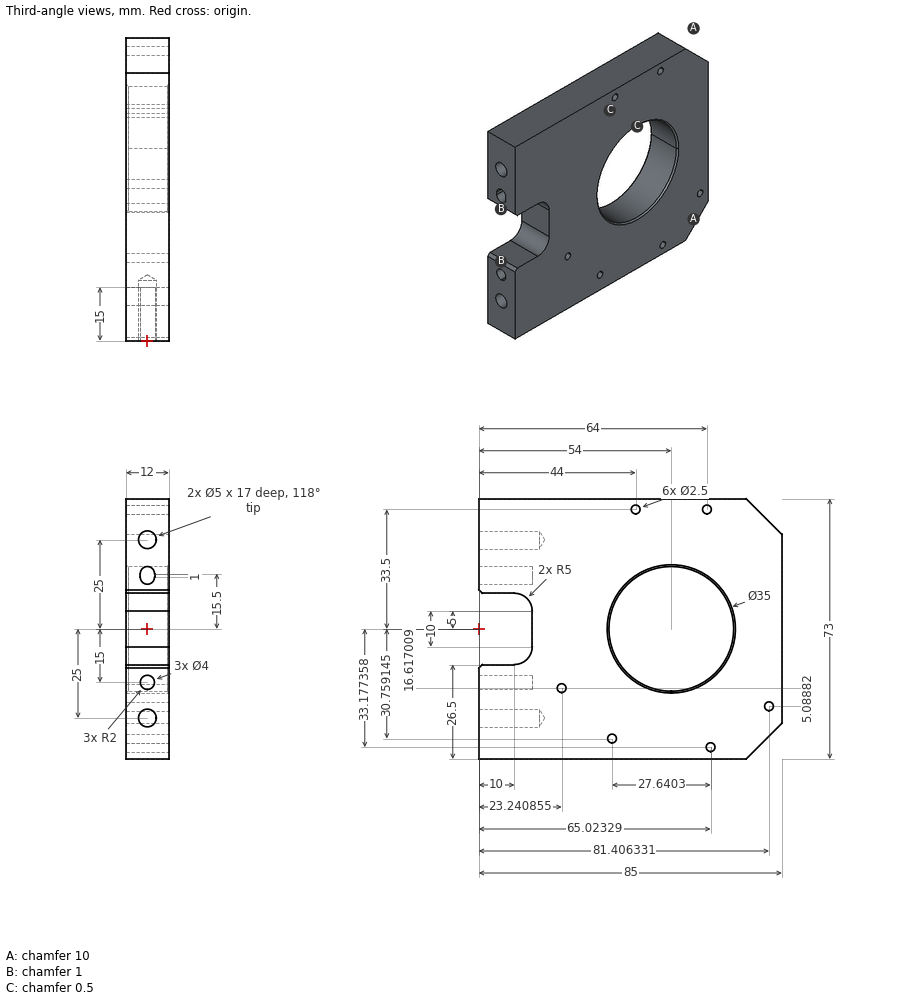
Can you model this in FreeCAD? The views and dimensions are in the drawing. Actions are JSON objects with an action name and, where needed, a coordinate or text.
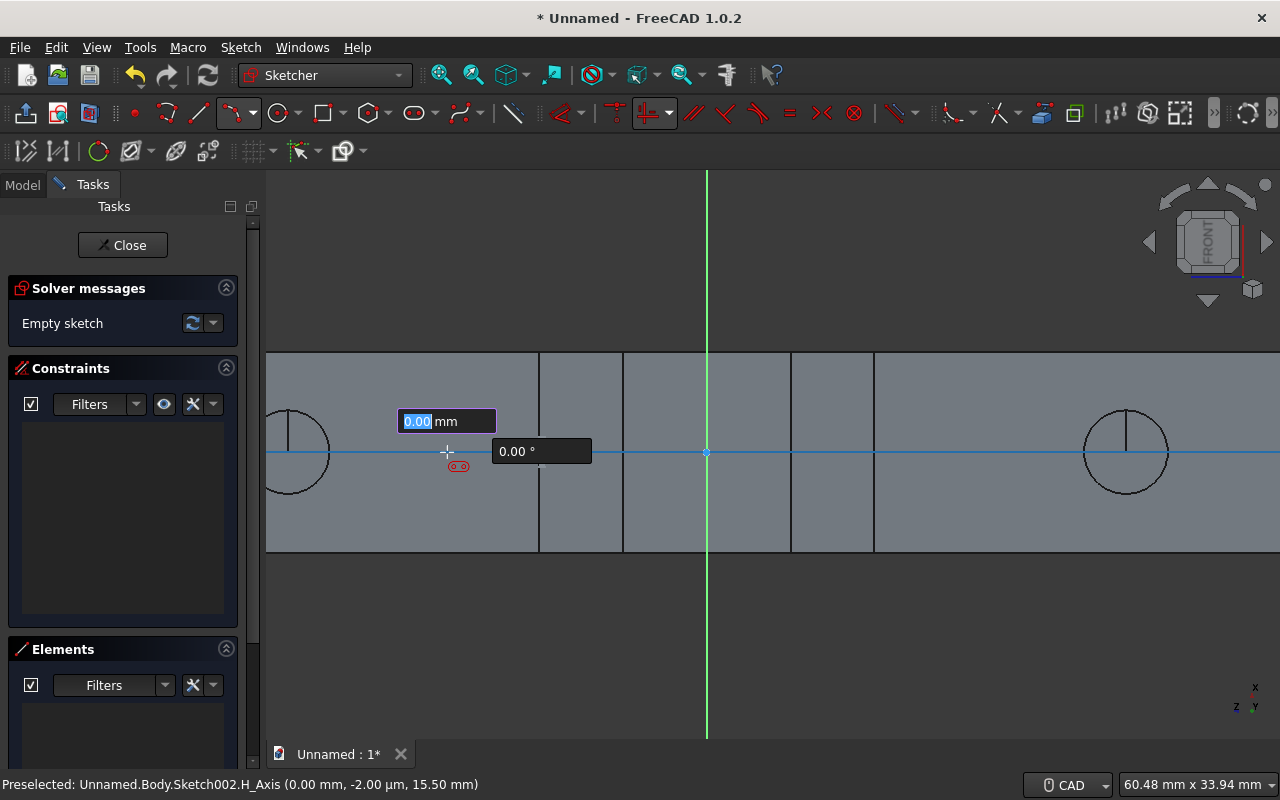
{"action": "left_click", "coordinate": [464, 443]}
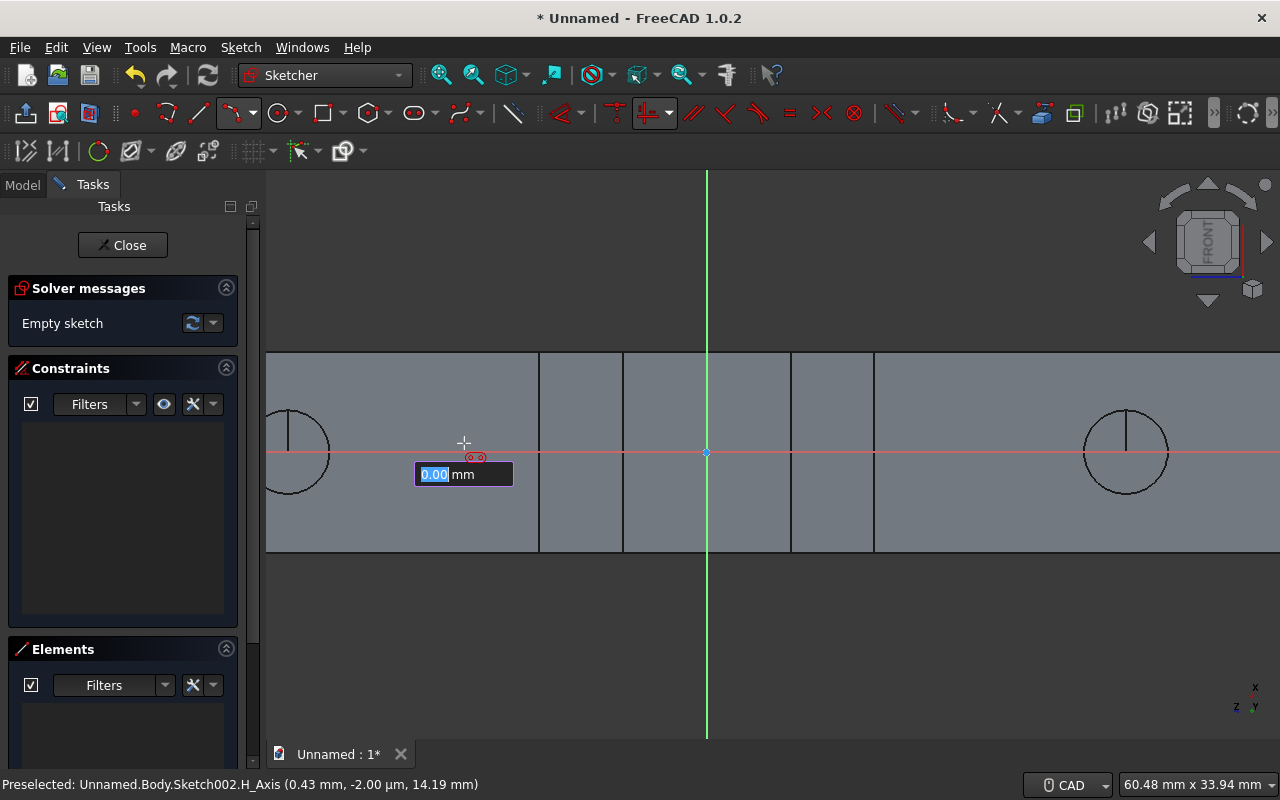
{"action": "left_click", "coordinate": [455, 419]}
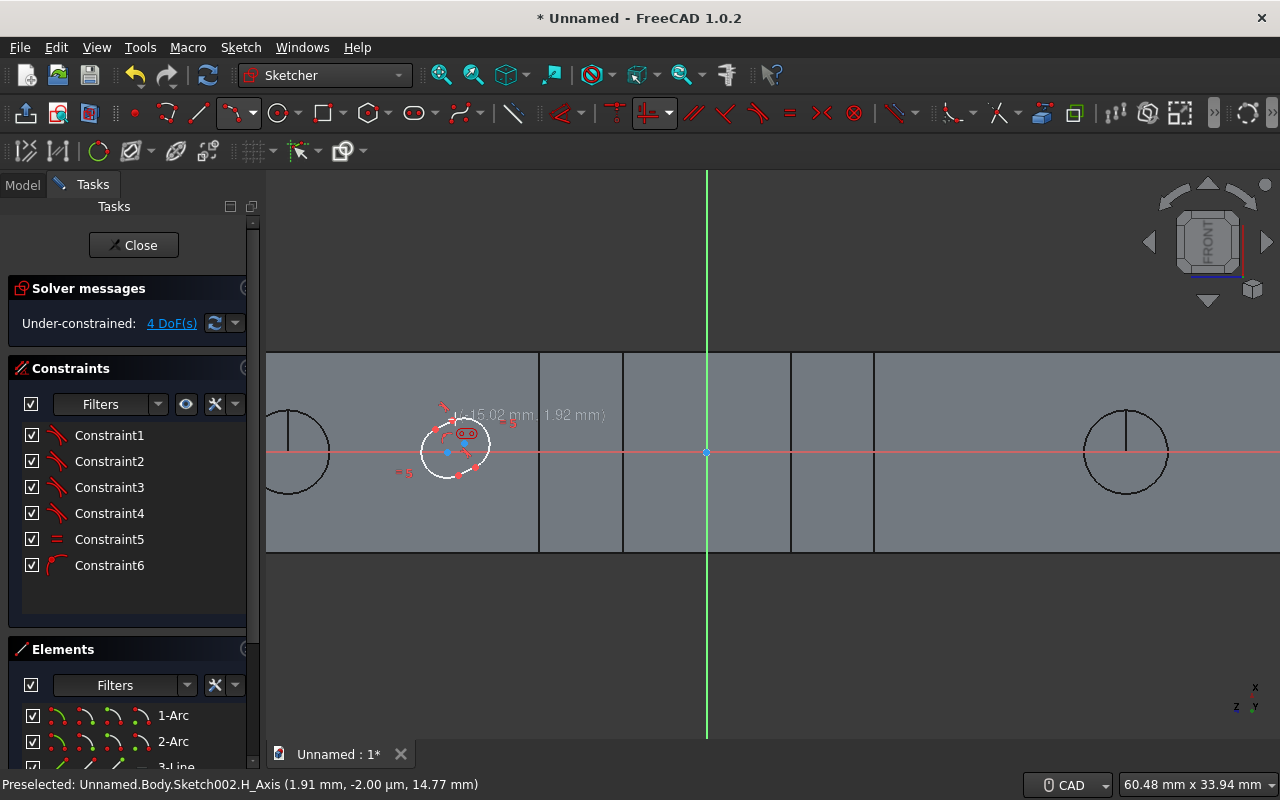
{"action": "left_click", "coordinate": [278, 114]}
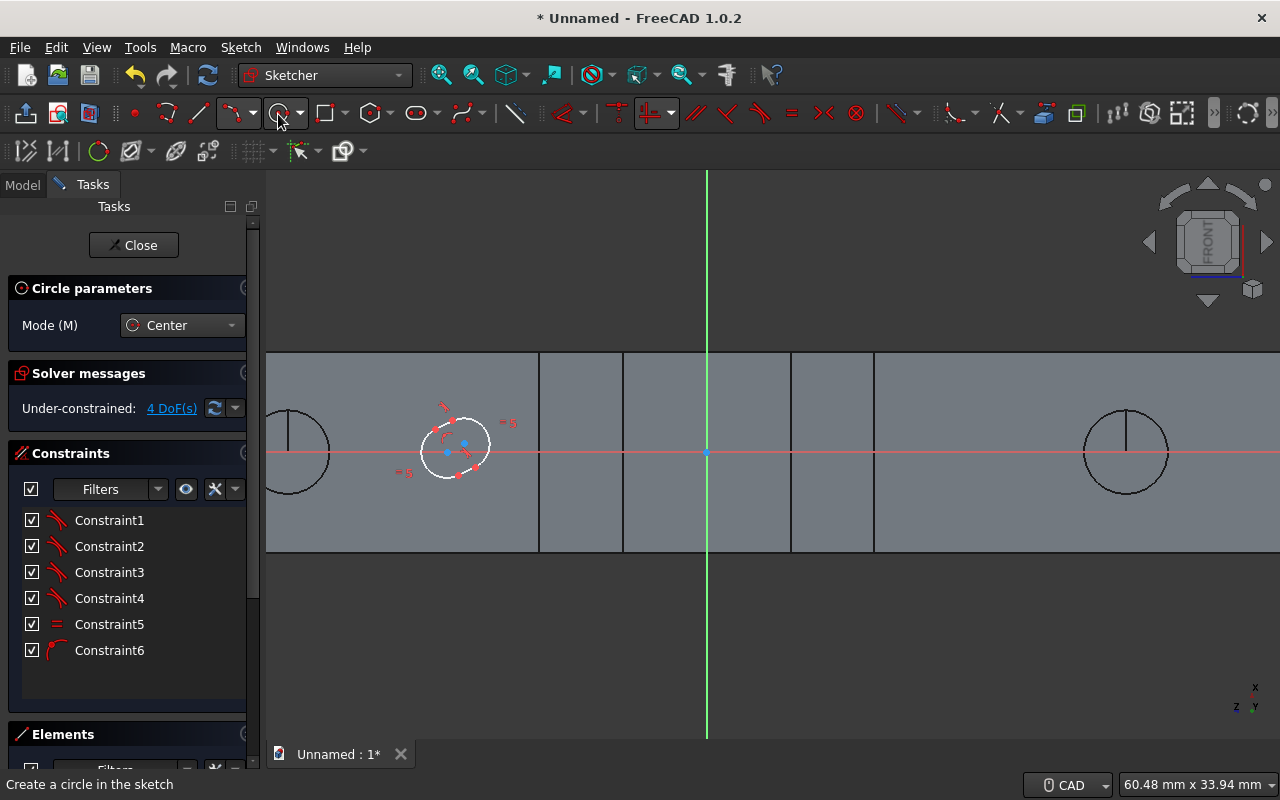
{"action": "left_click", "coordinate": [958, 452]}
{"action": "mouse_move", "coordinate": [982, 428]}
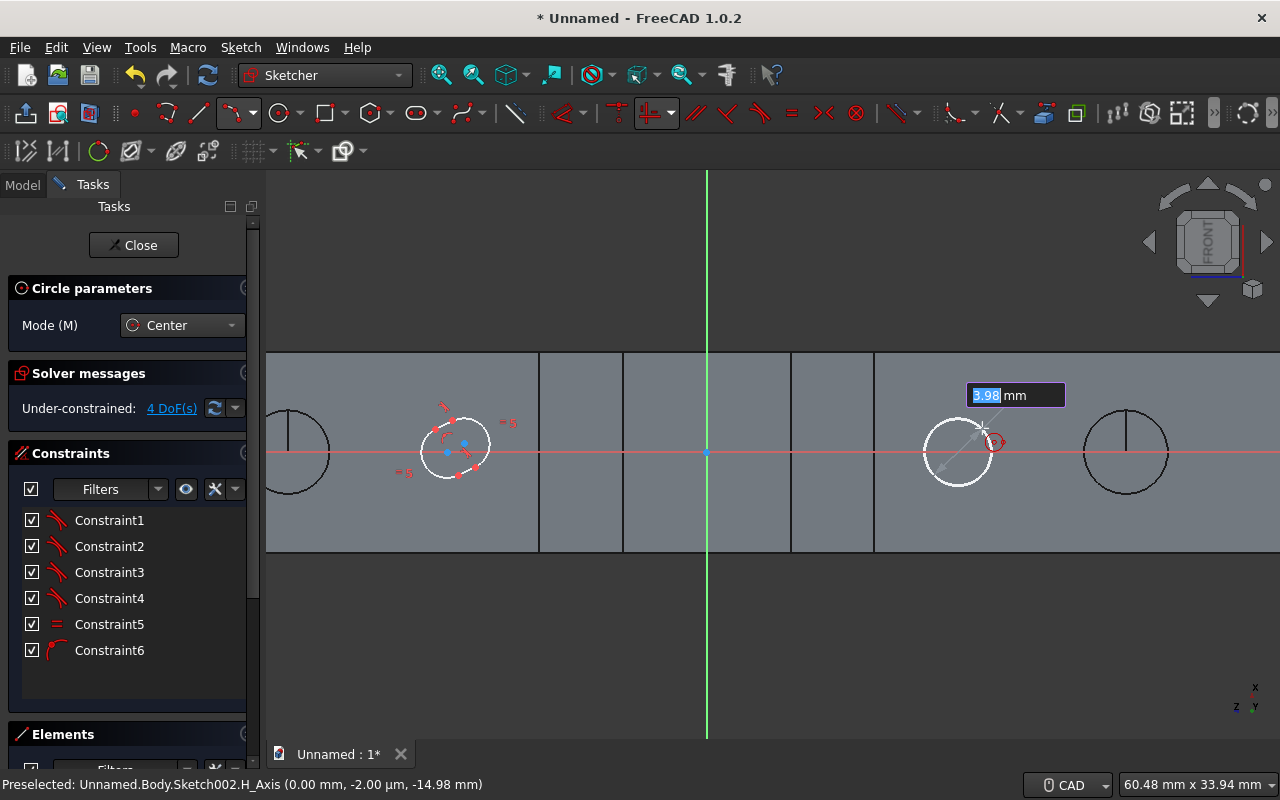
{"action": "type", "text": "4"}
{"action": "key", "text": "Return"}
{"action": "key", "text": "Escape"}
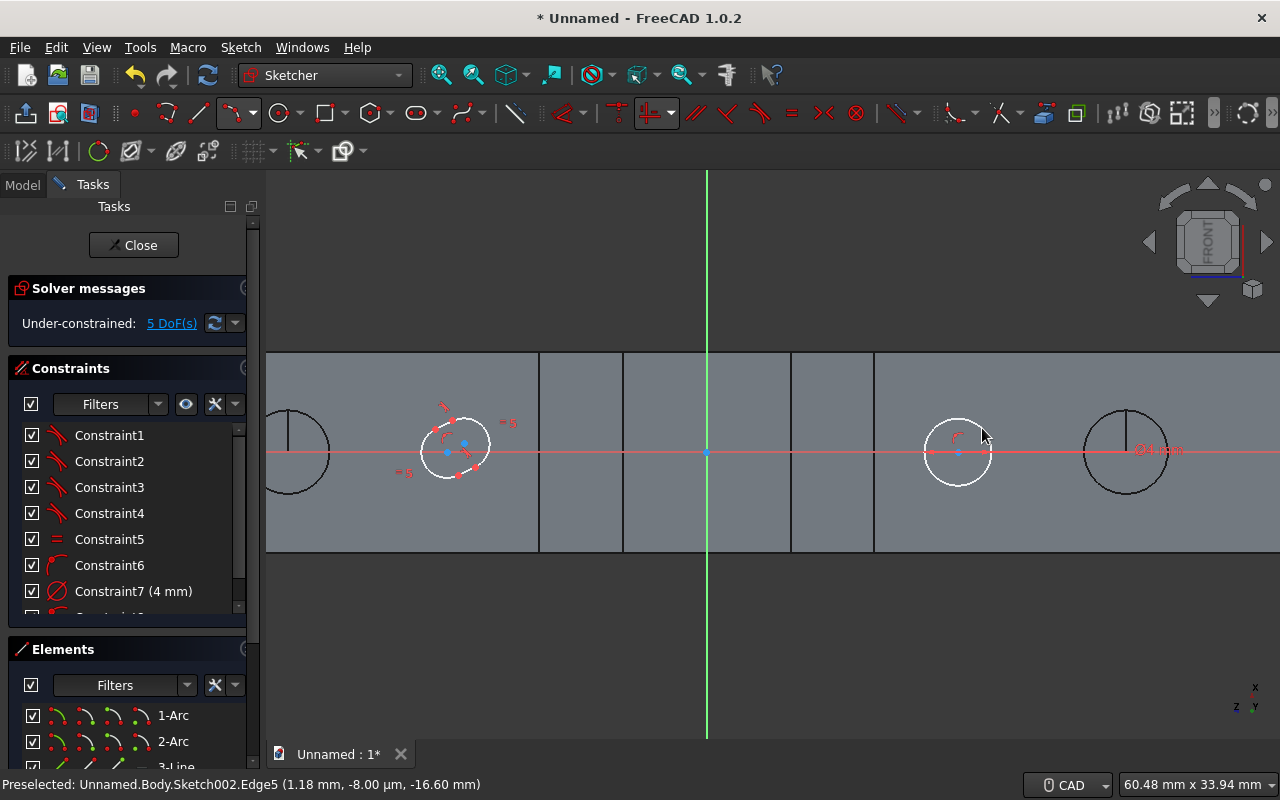
{"action": "left_click", "coordinate": [464, 444]}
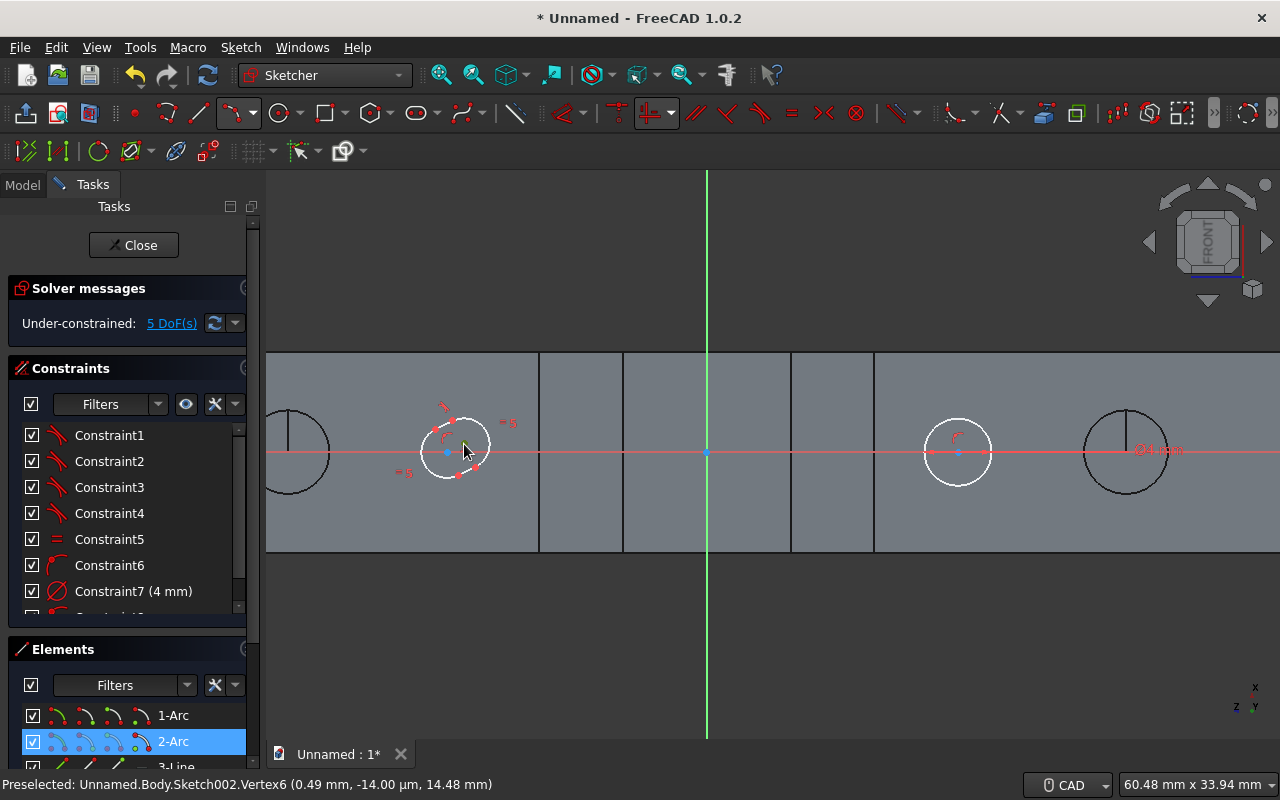
{"action": "left_click", "coordinate": [353, 452]}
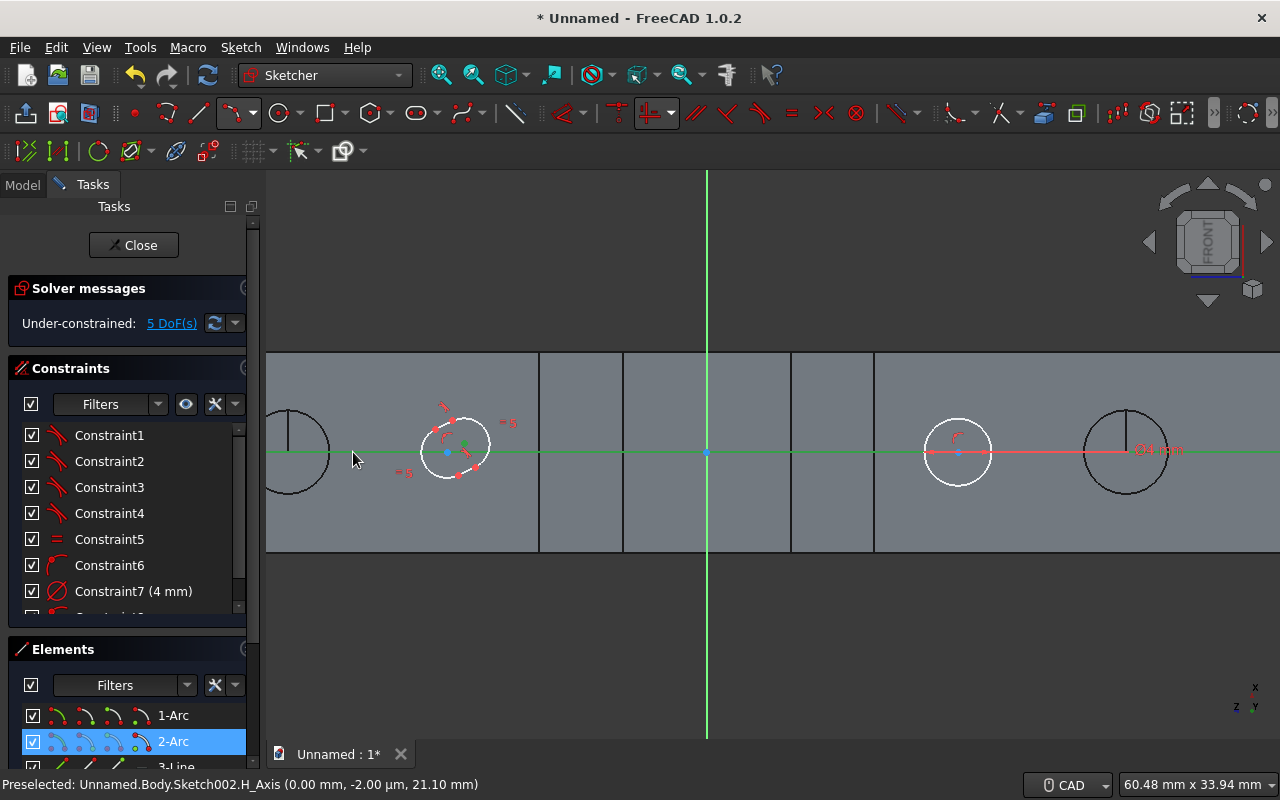
{"action": "left_click", "coordinate": [618, 114]}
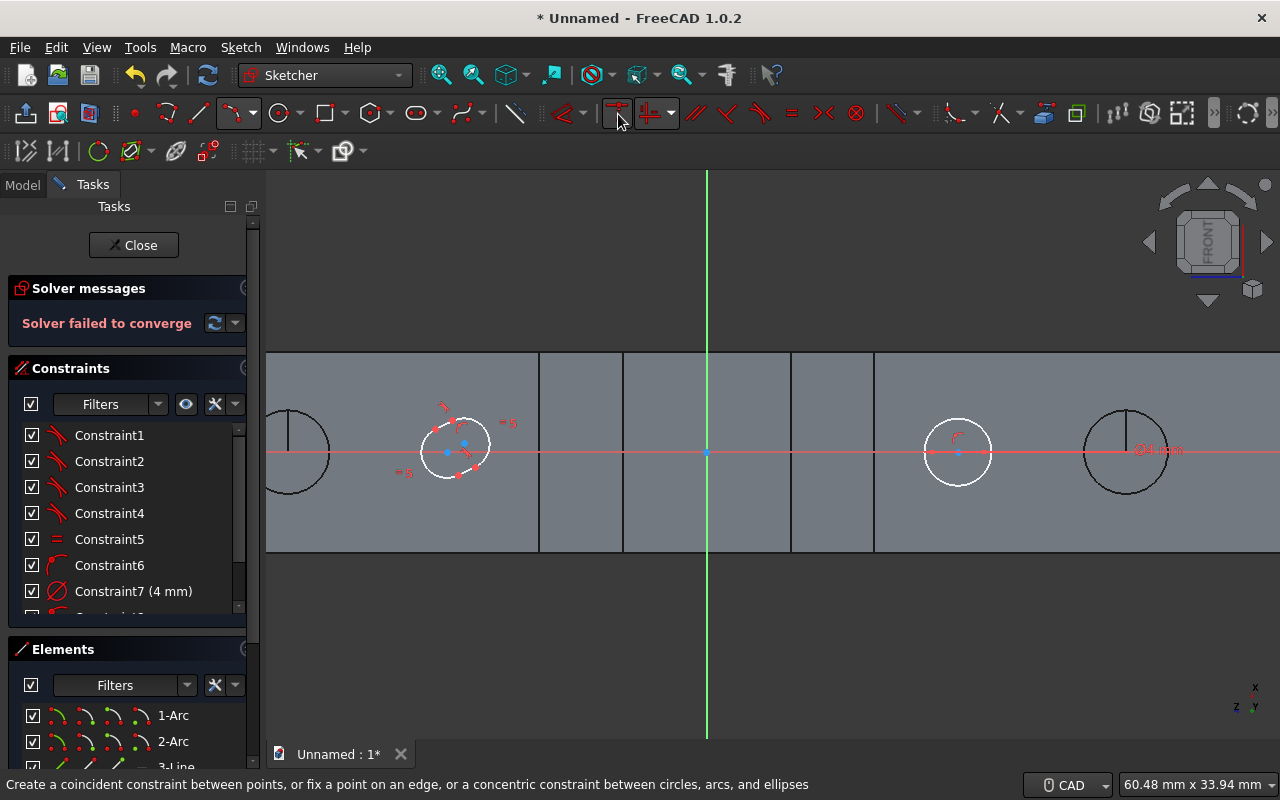
{"action": "left_click", "coordinate": [562, 114]}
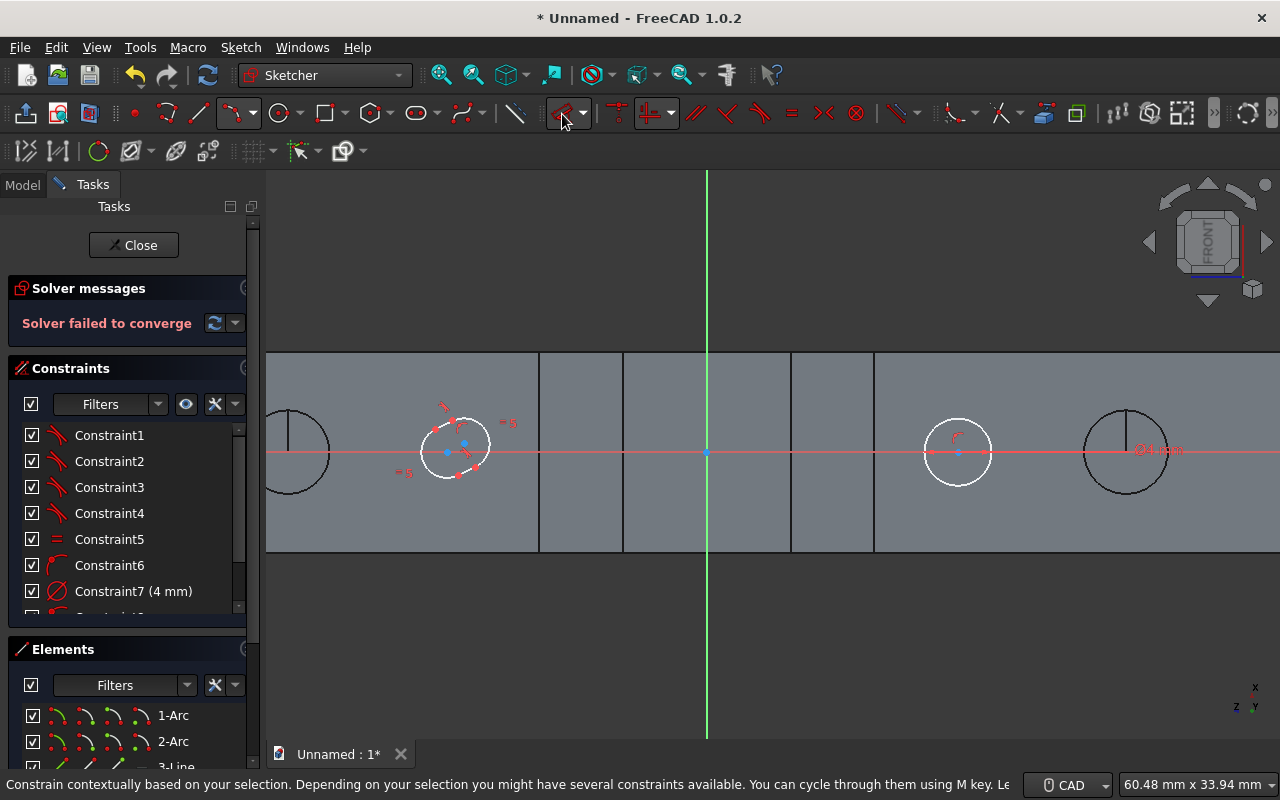
{"action": "left_click", "coordinate": [435, 475]}
{"action": "left_click", "coordinate": [420, 503]}